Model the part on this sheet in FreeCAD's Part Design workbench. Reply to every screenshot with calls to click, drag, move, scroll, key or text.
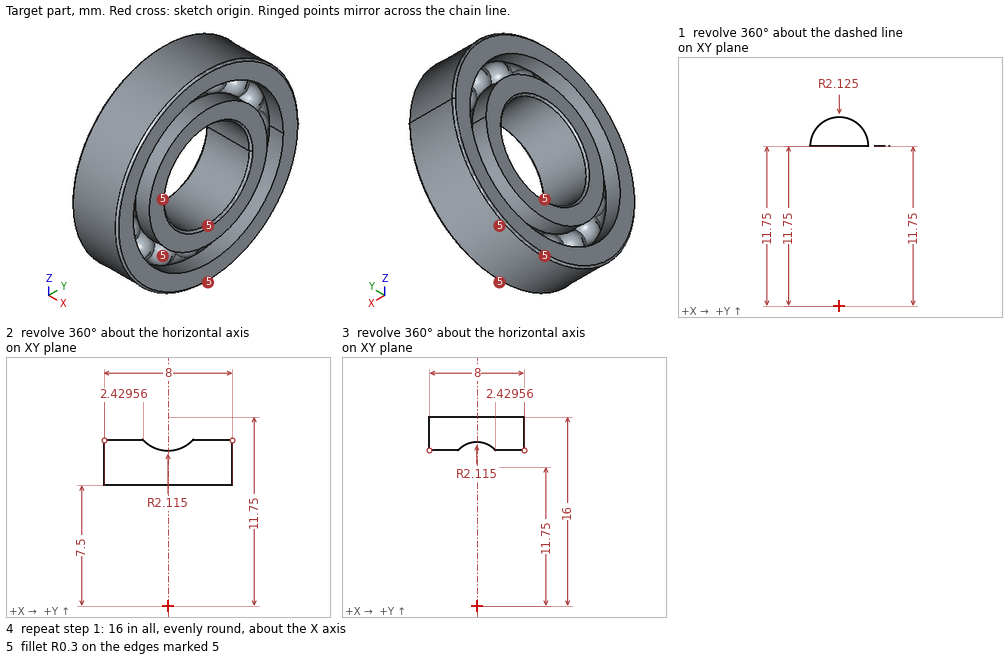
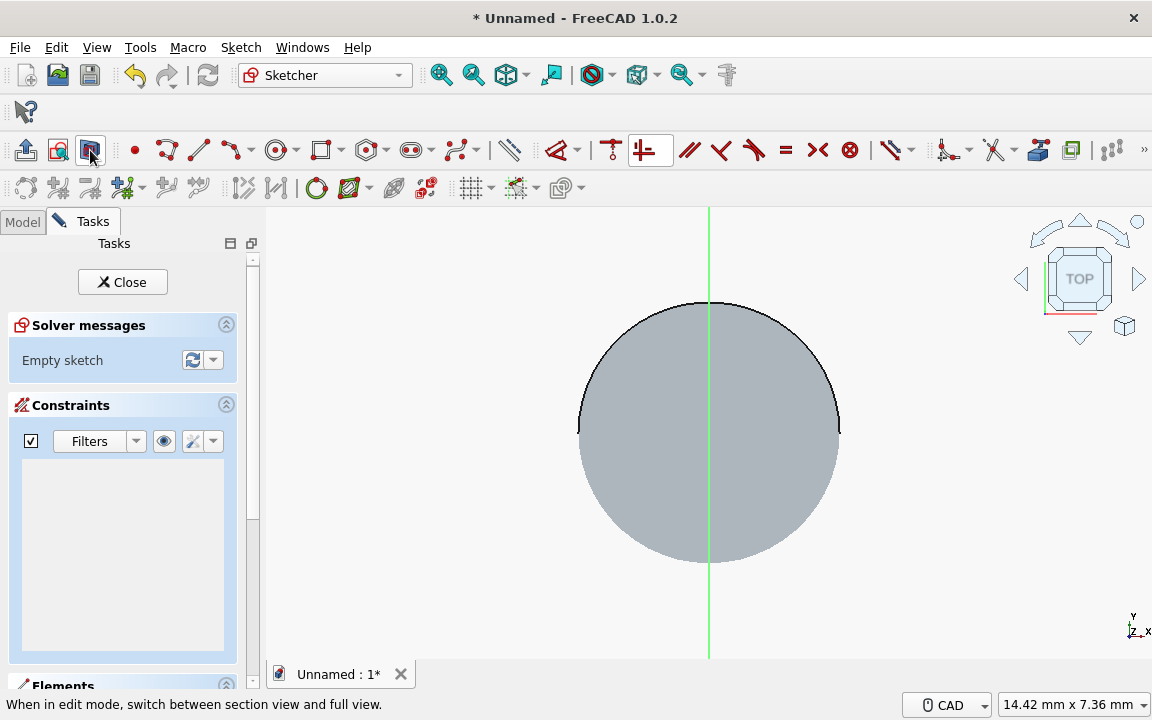
scroll(601, 235, down, 5)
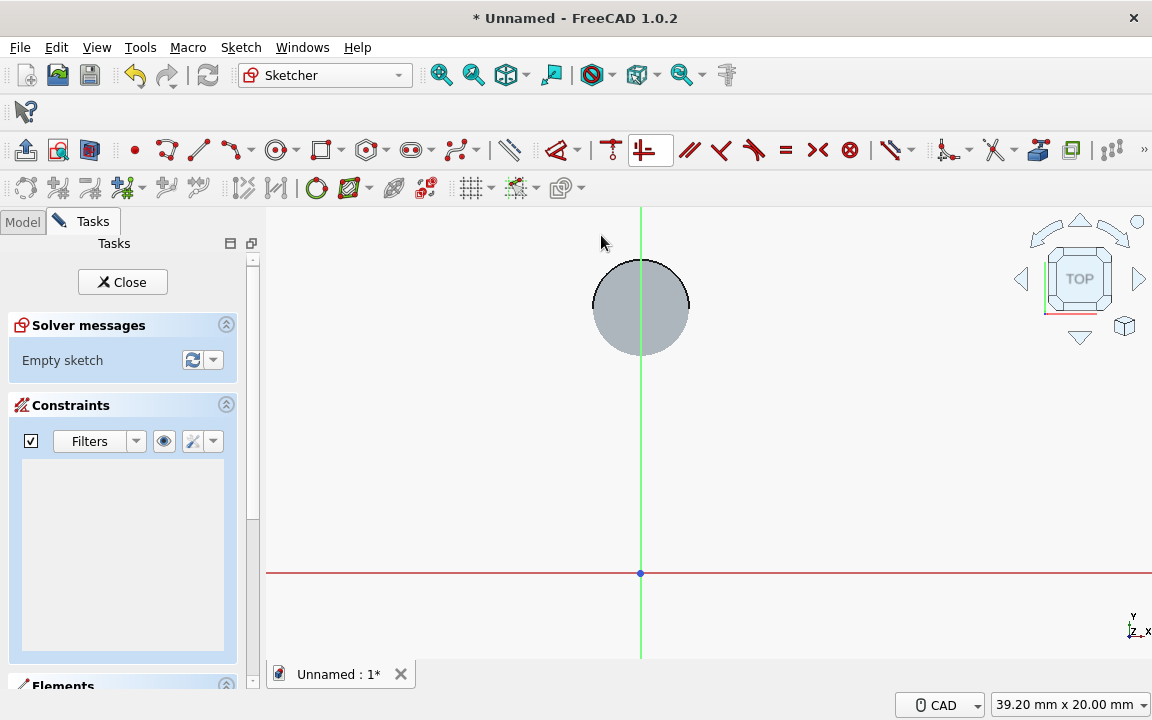
click(168, 150)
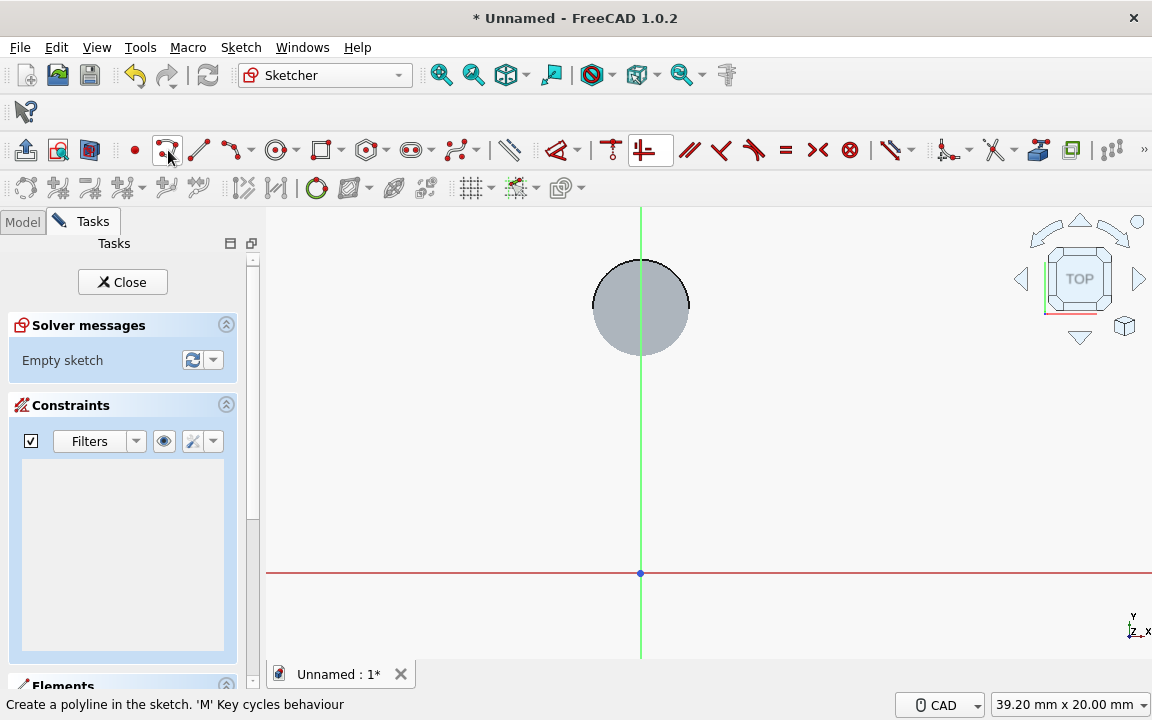
click(605, 340)
click(551, 340)
click(551, 404)
click(731, 404)
click(731, 340)
click(676, 340)
right_click(676, 340)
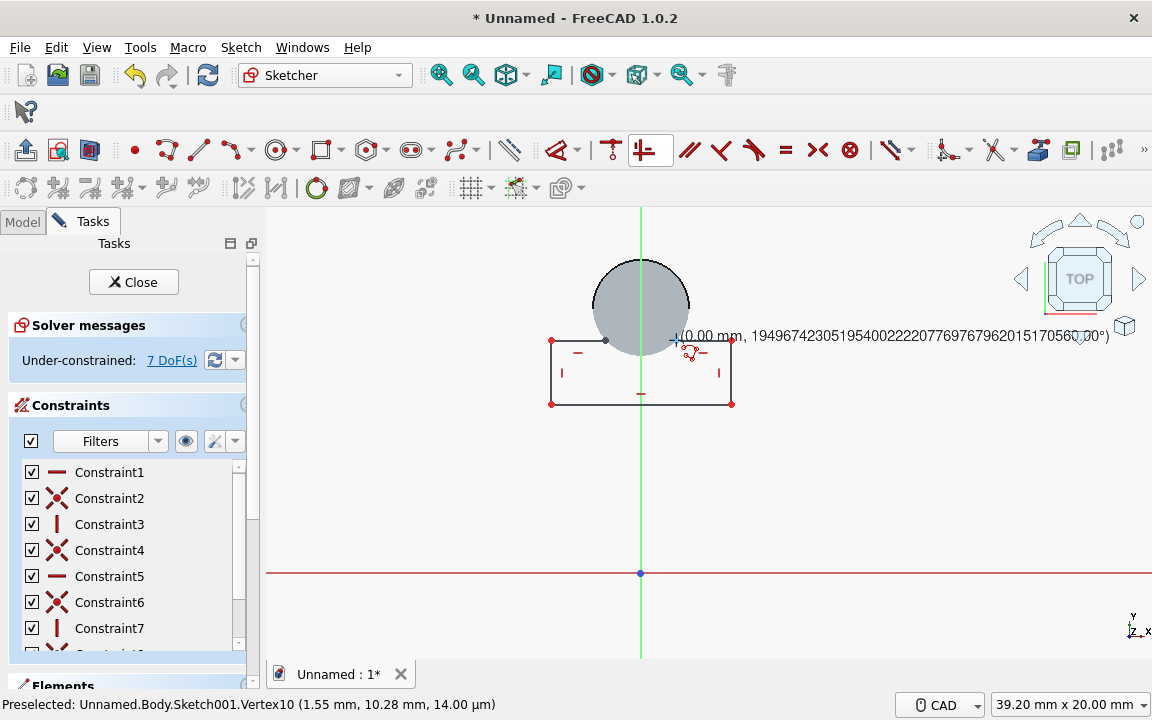
click(232, 150)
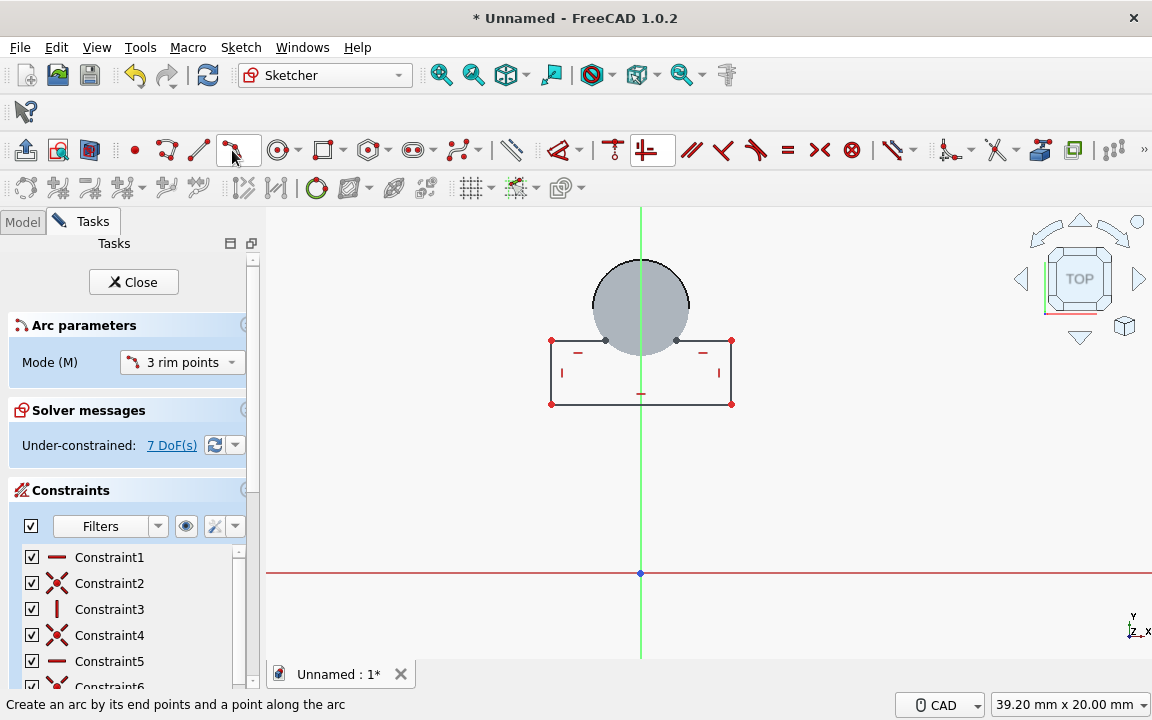
click(676, 341)
click(605, 341)
click(625, 353)
key(Escape)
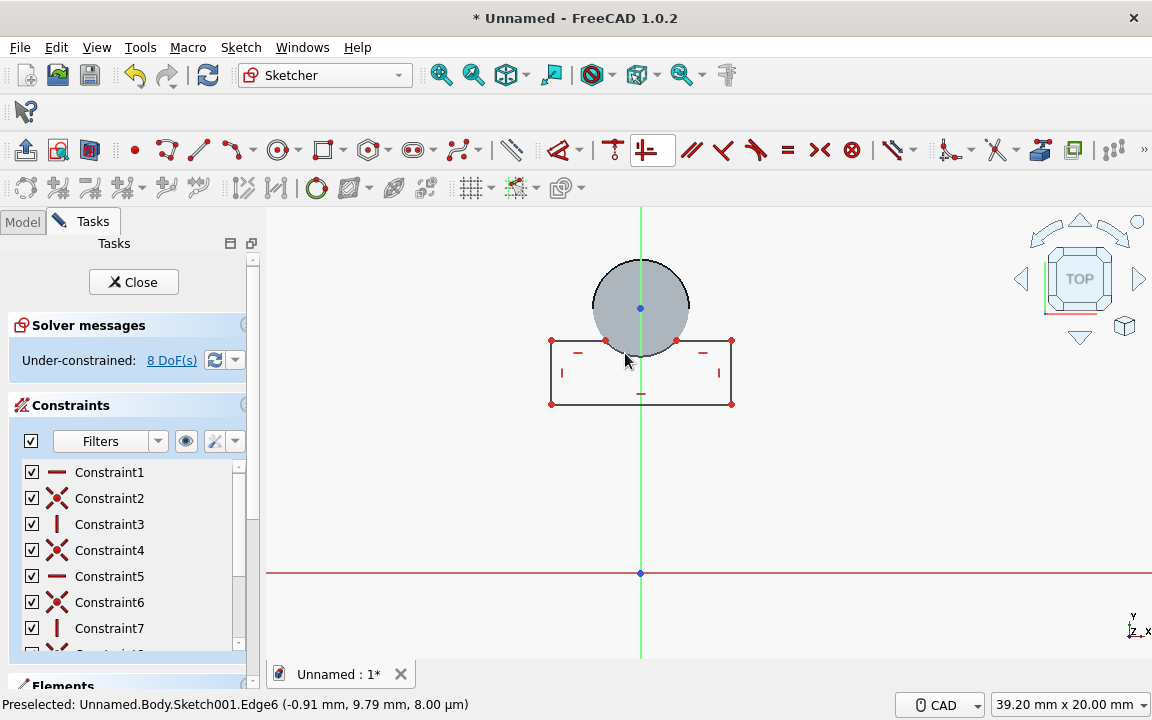
click(641, 308)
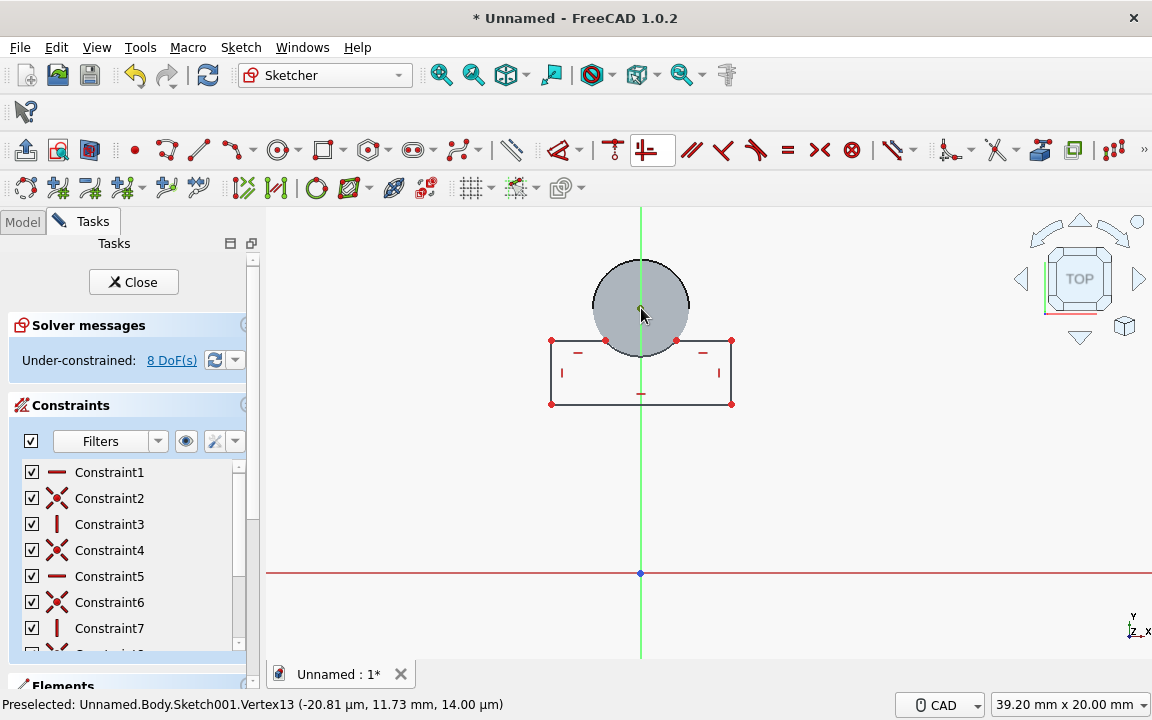
click(641, 518)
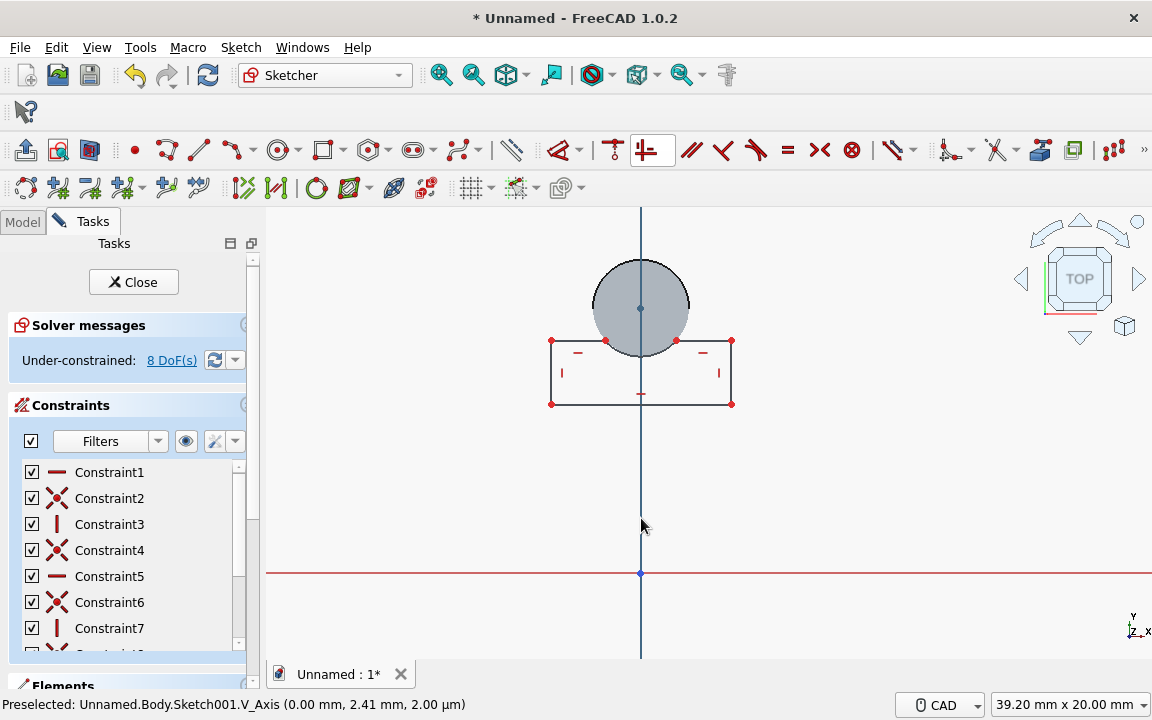
click(614, 150)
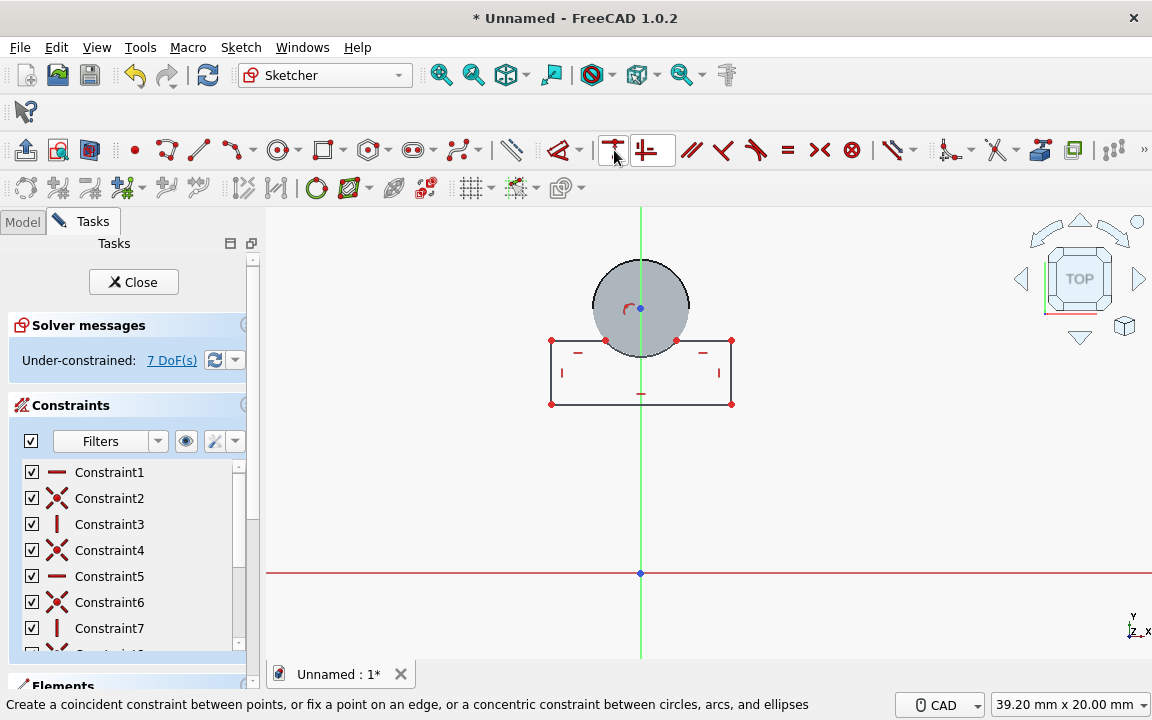
click(551, 341)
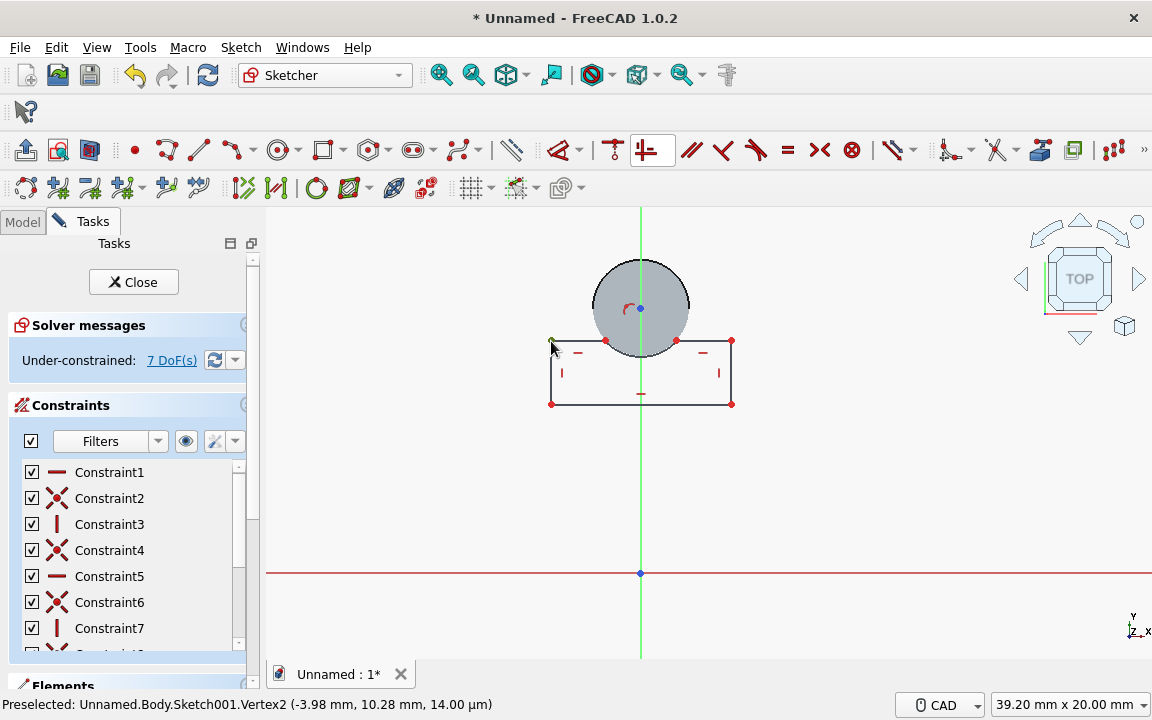
click(731, 341)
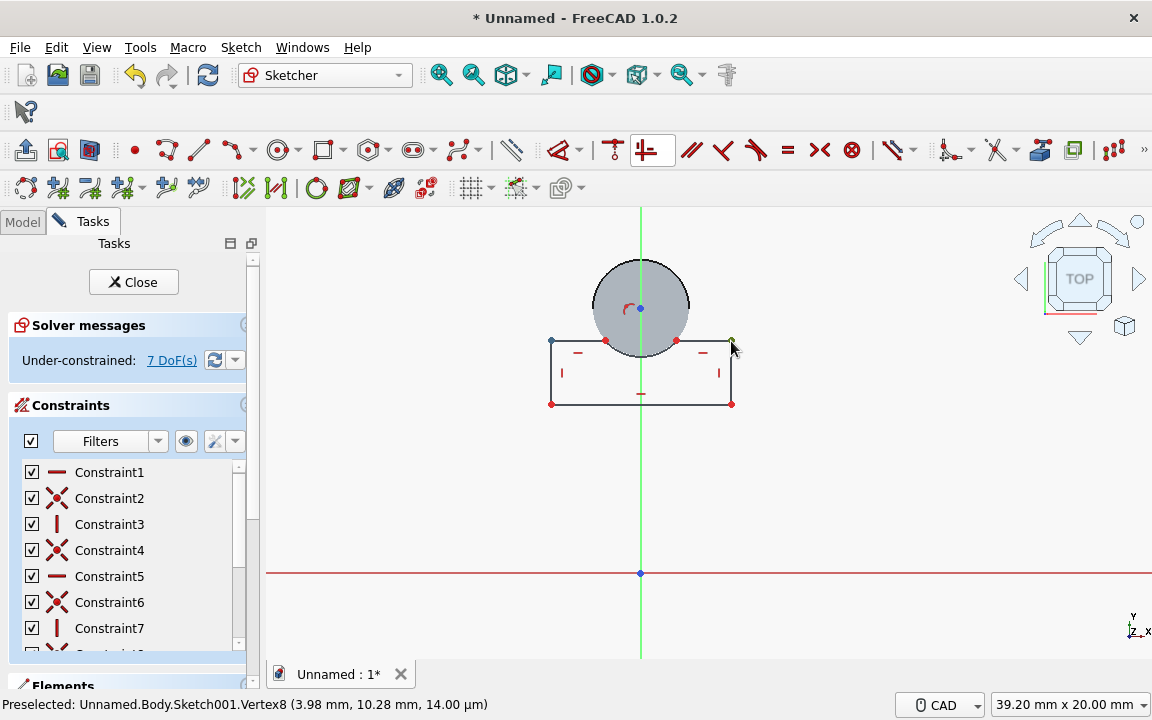
click(641, 518)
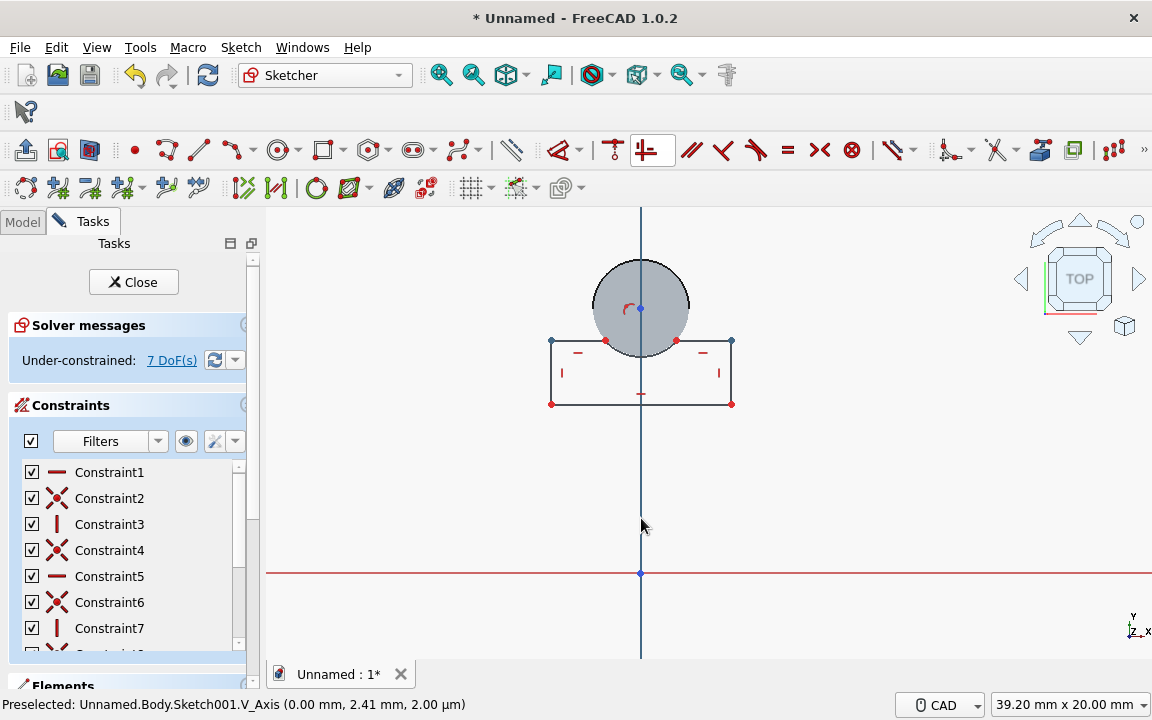
click(820, 150)